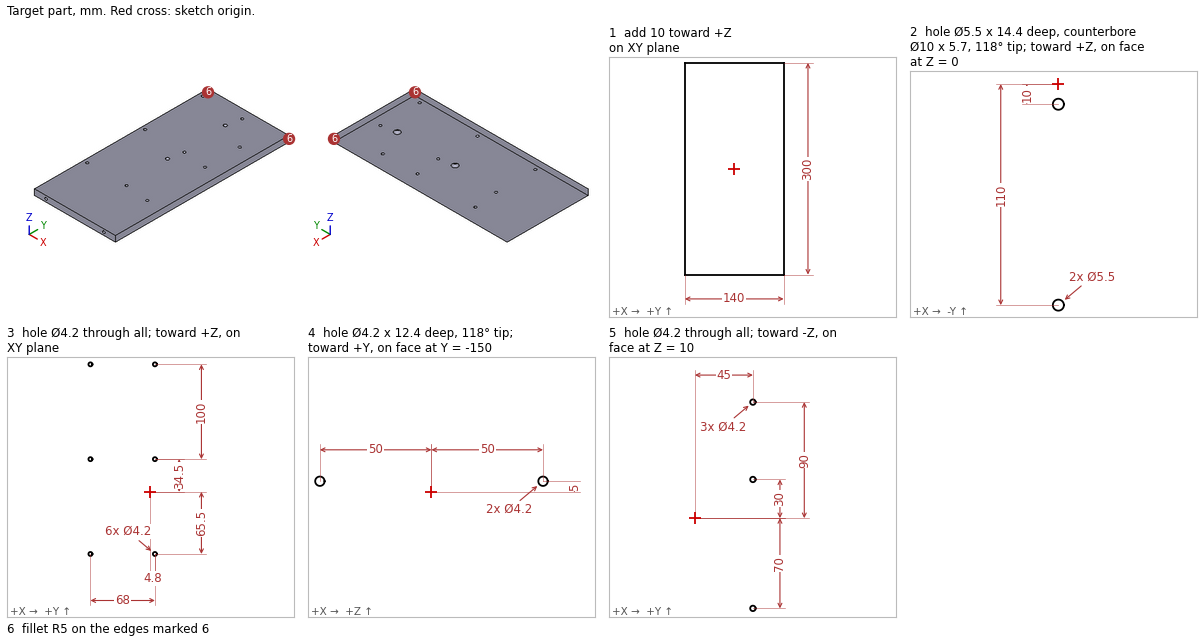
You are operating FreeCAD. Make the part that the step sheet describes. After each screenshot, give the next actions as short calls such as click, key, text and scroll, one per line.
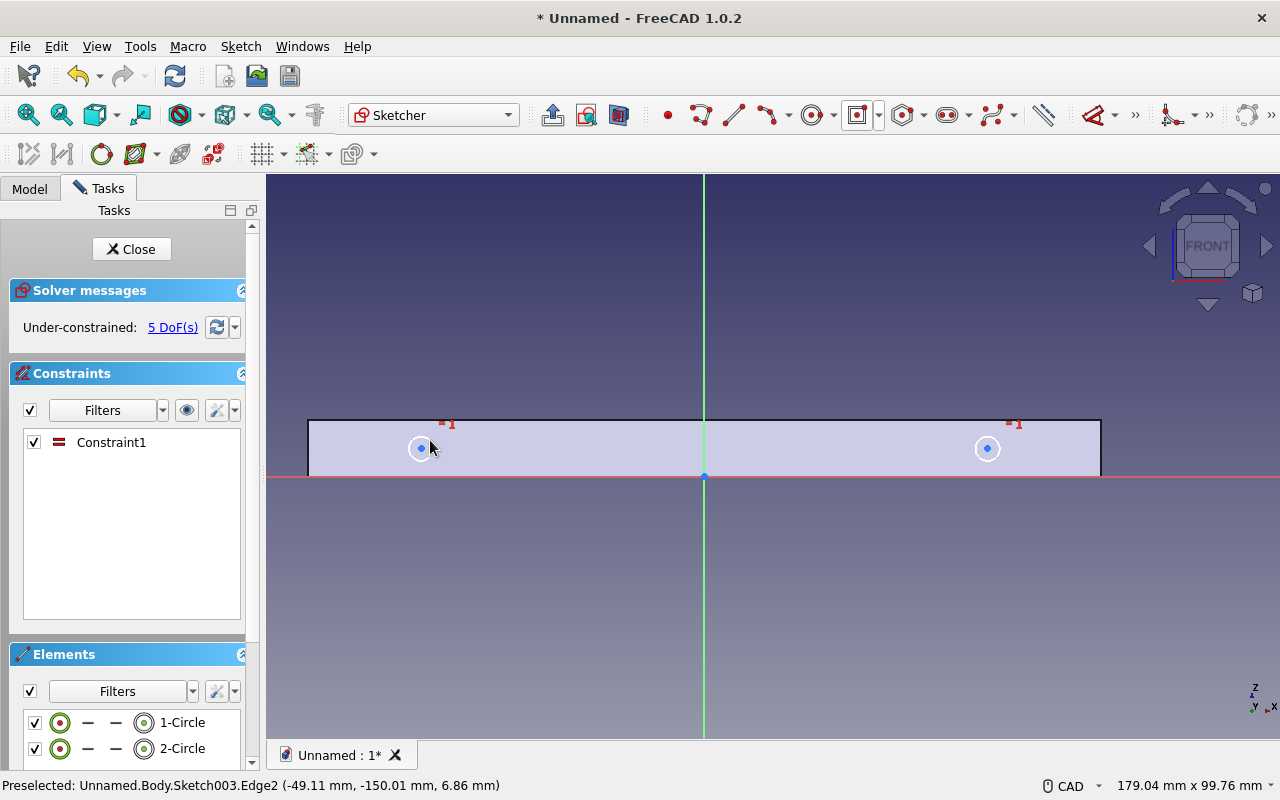
click(988, 449)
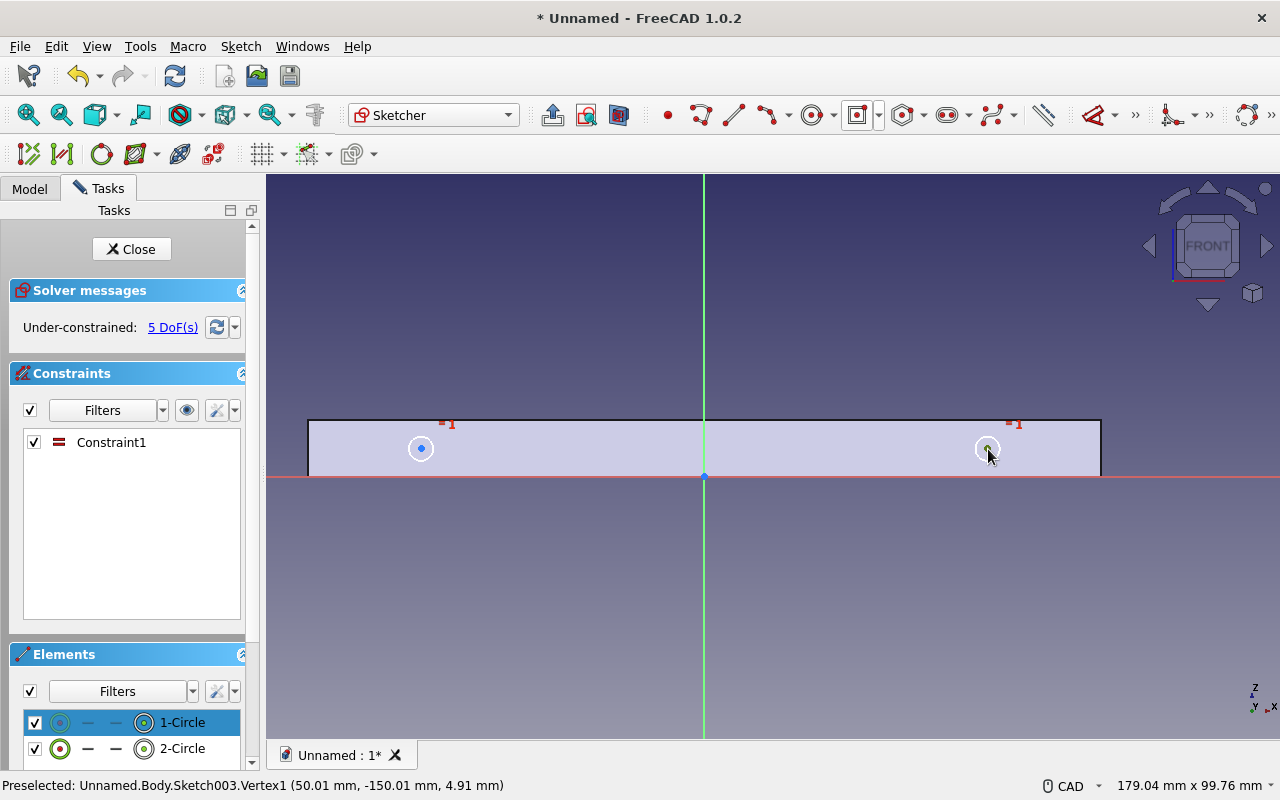
click(421, 449)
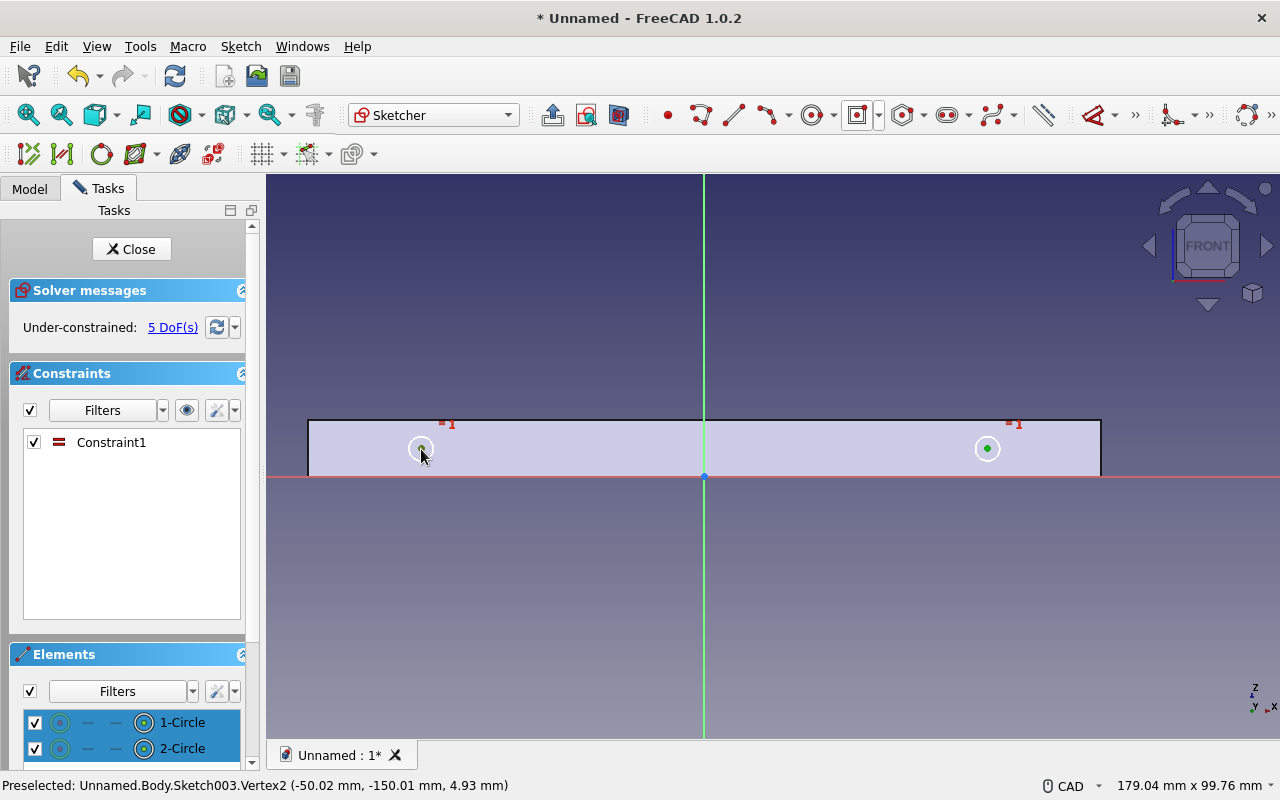
key(h)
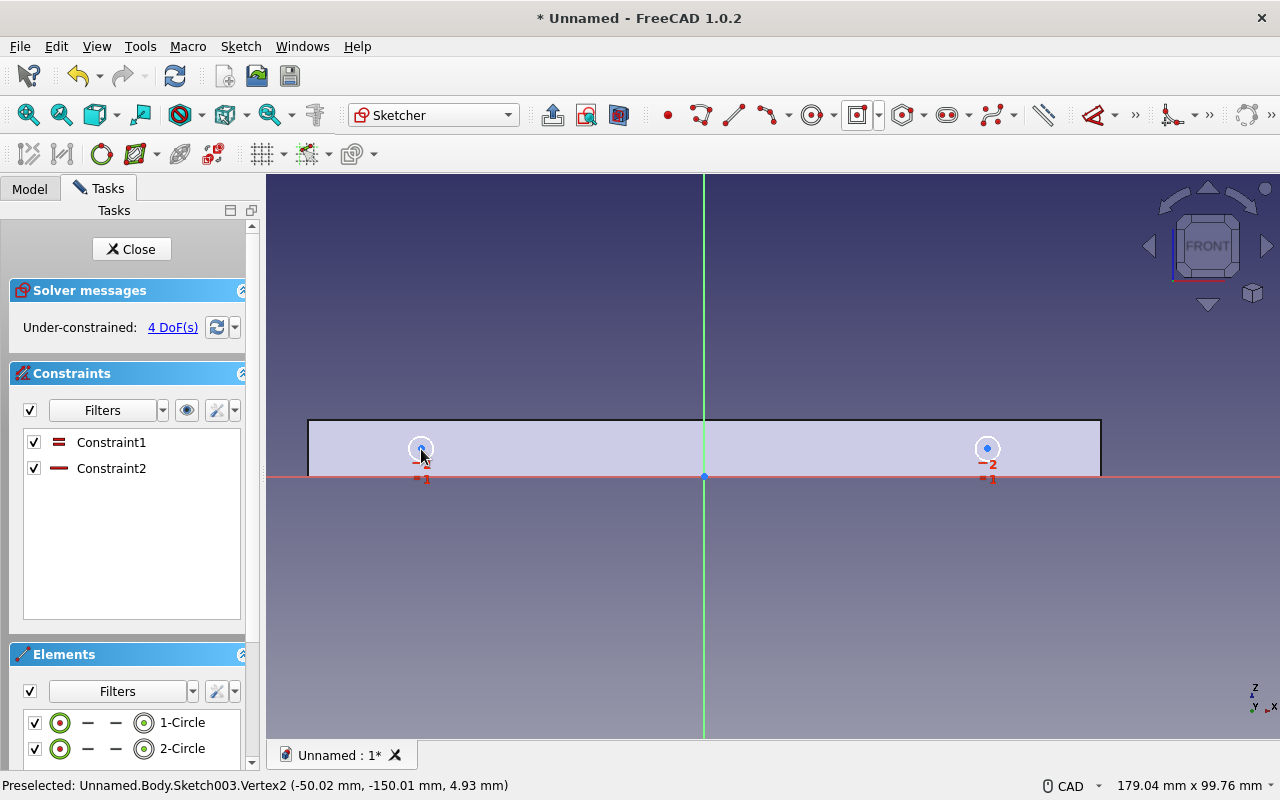
key(d)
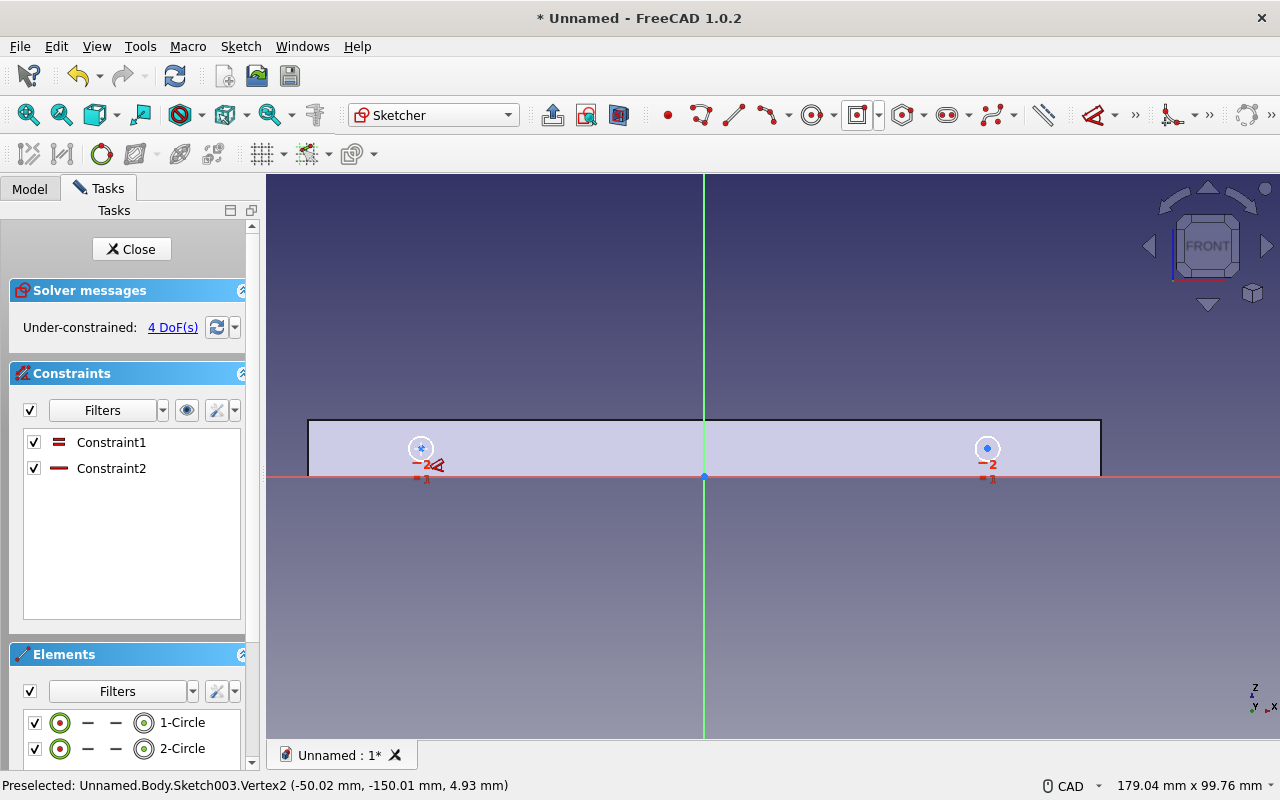
scroll(996, 440, up, 3)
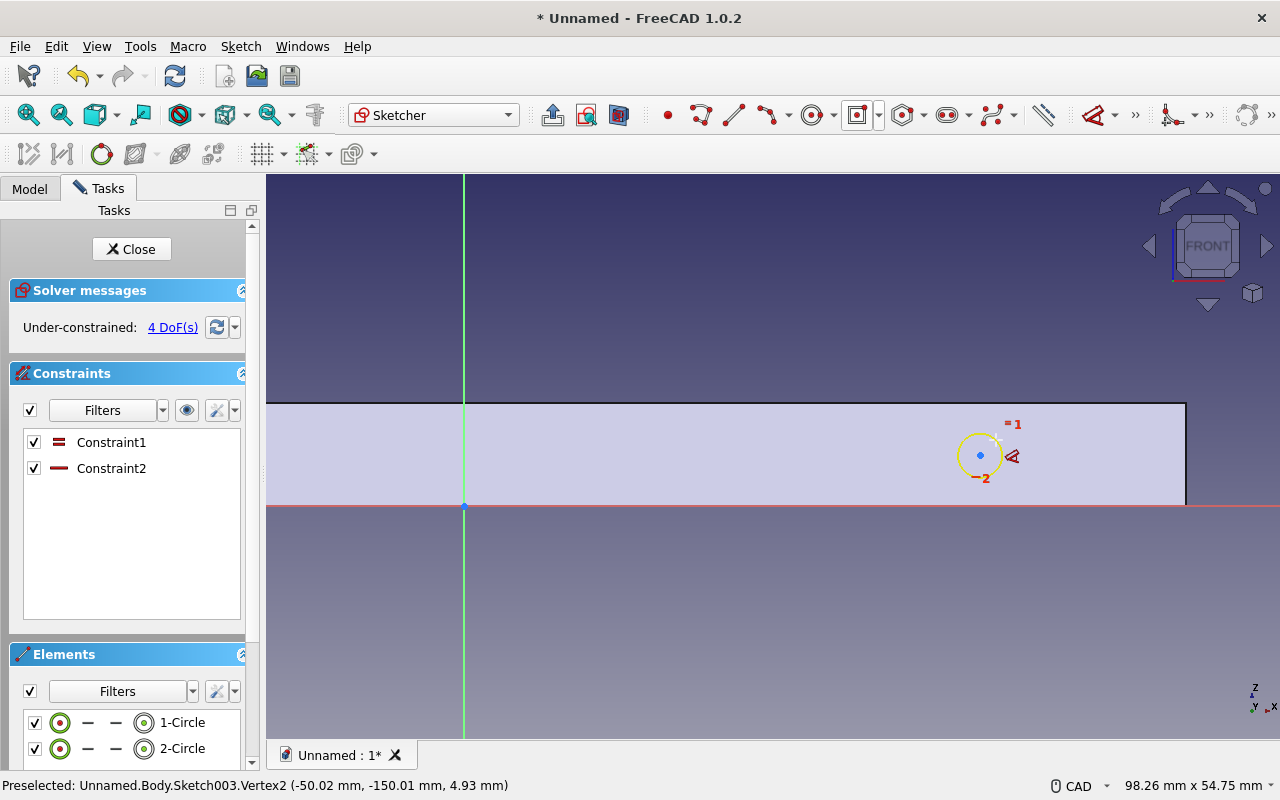
click(996, 440)
click(1019, 418)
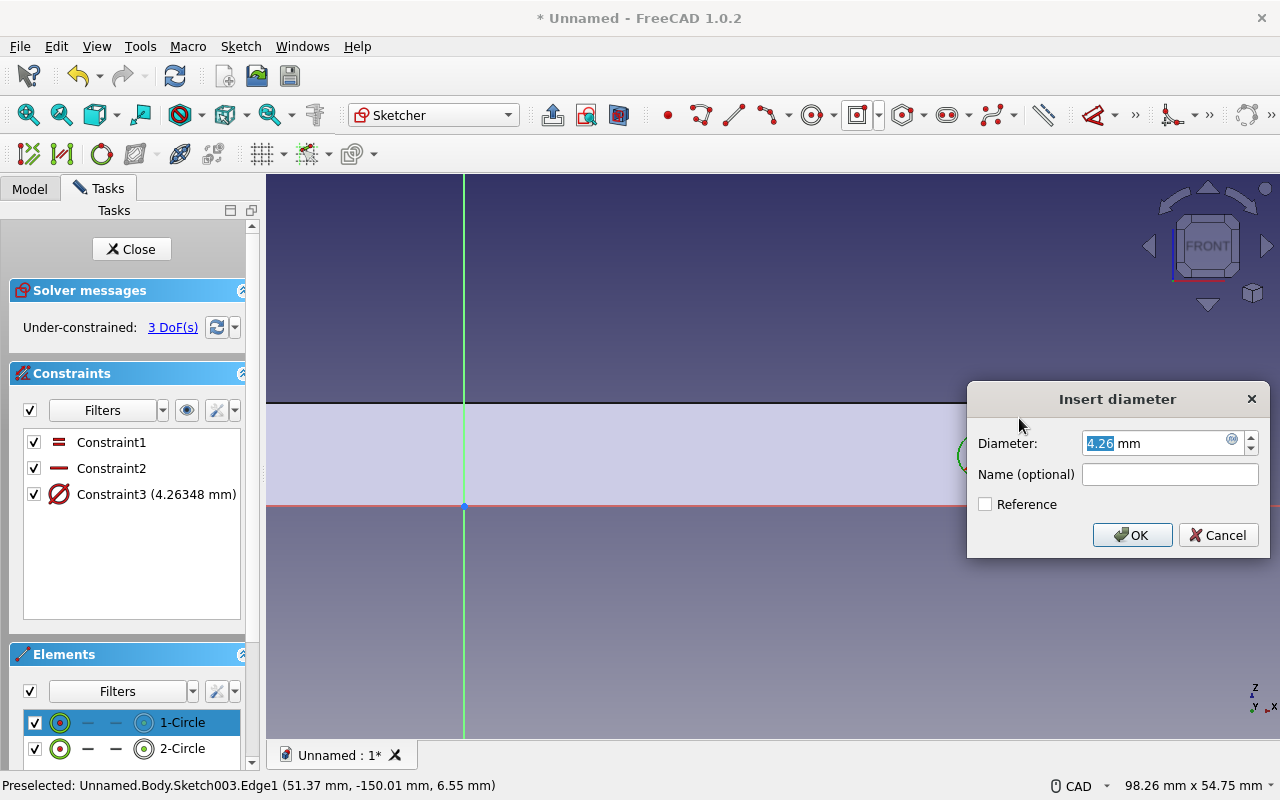
text(4.2)
key(Return)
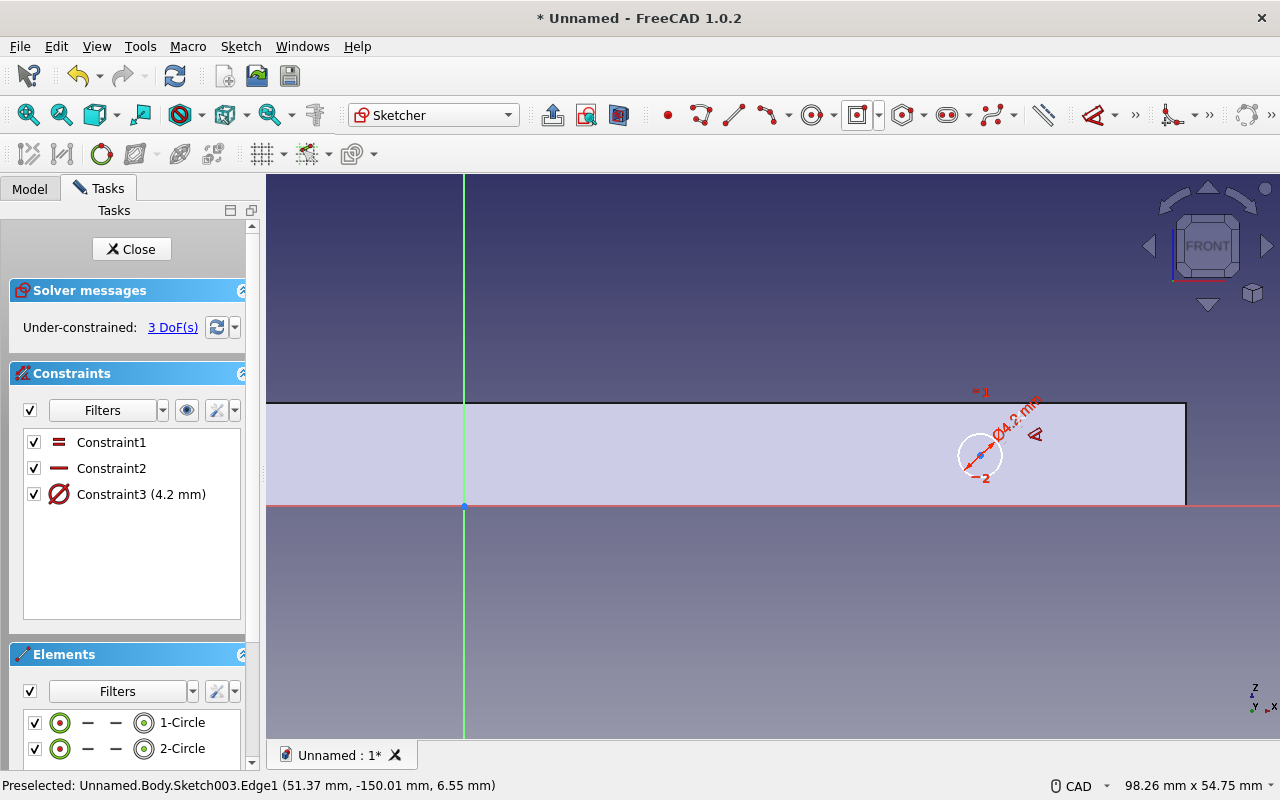
click(980, 456)
click(1014, 481)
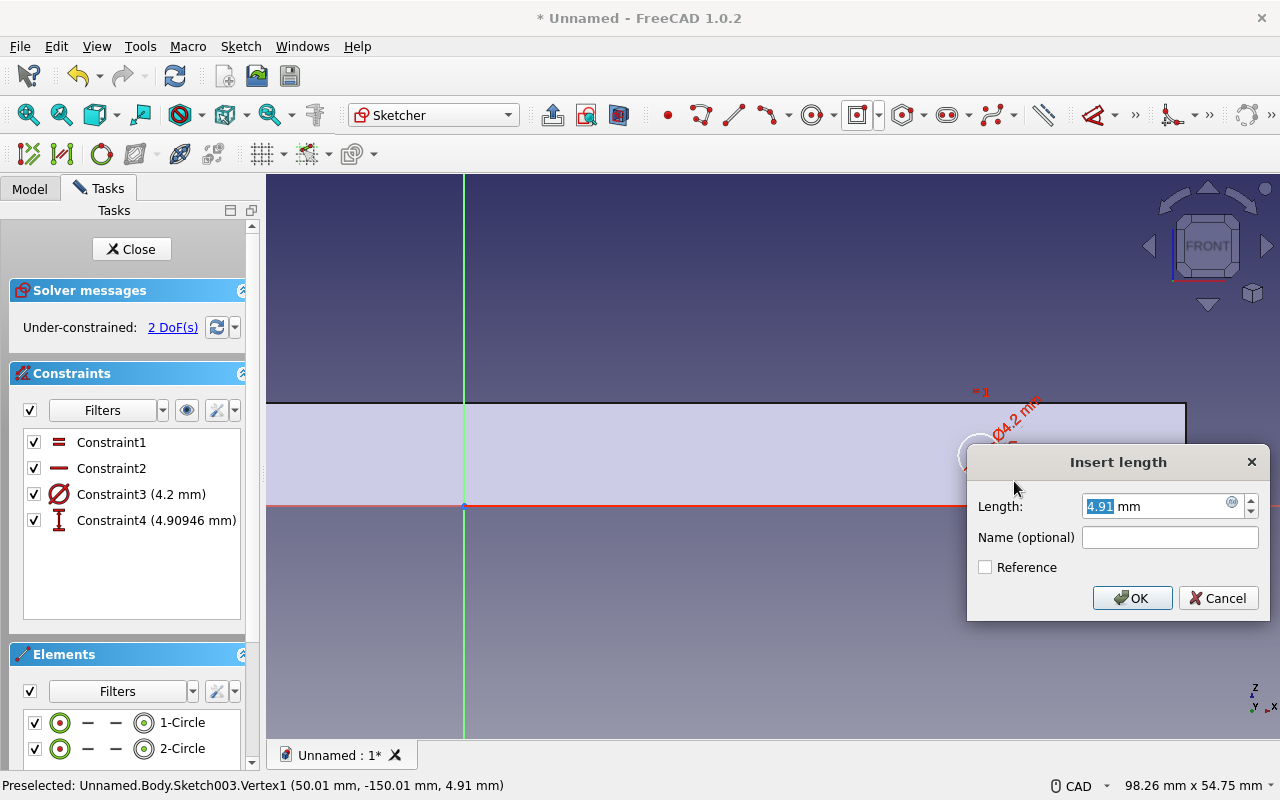
text(5)
key(Return)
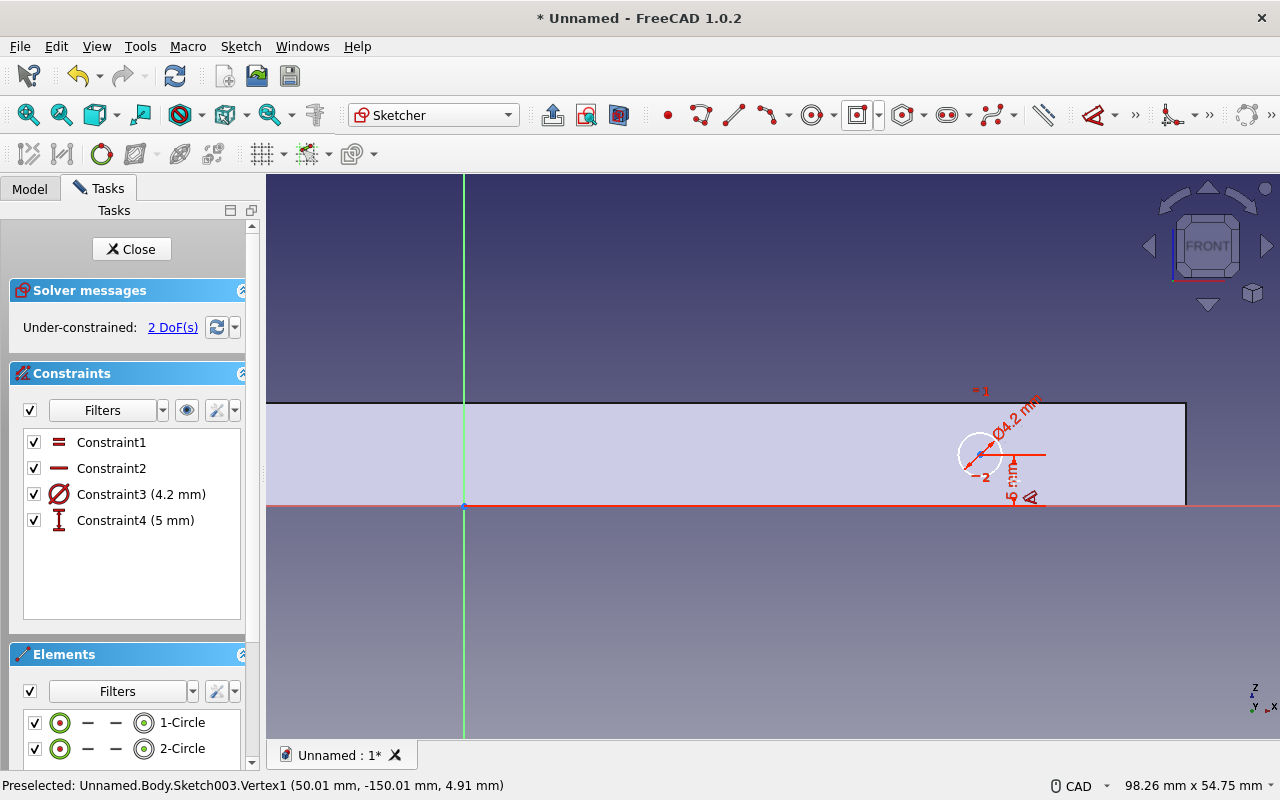
click(980, 455)
click(722, 540)